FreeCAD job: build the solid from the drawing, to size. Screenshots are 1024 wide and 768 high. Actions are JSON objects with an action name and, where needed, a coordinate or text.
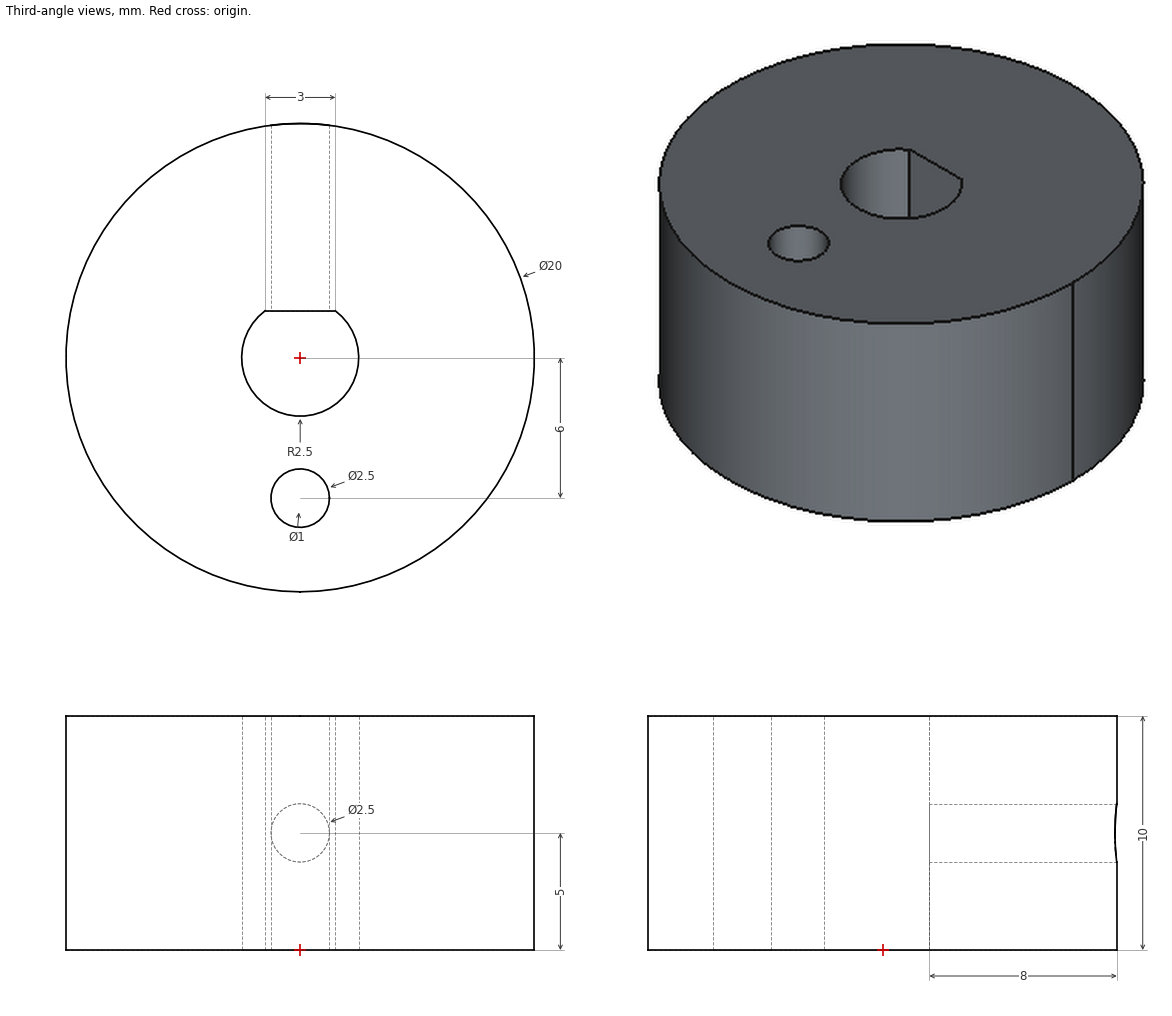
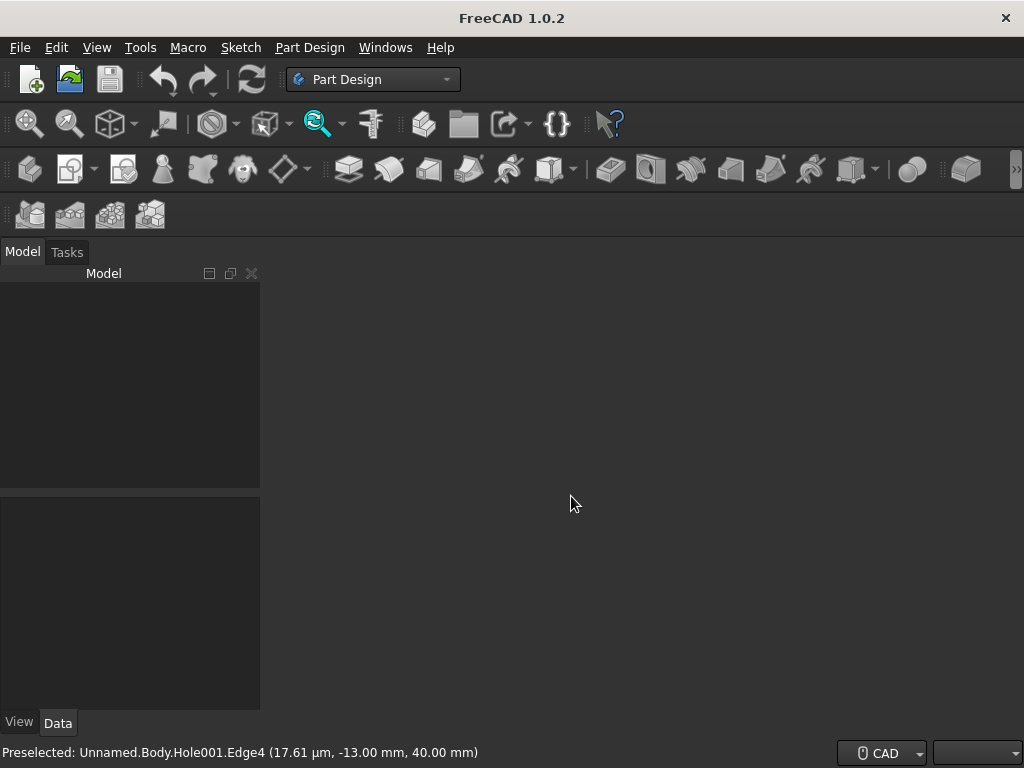
{"action": "left_click", "coordinate": [30, 80]}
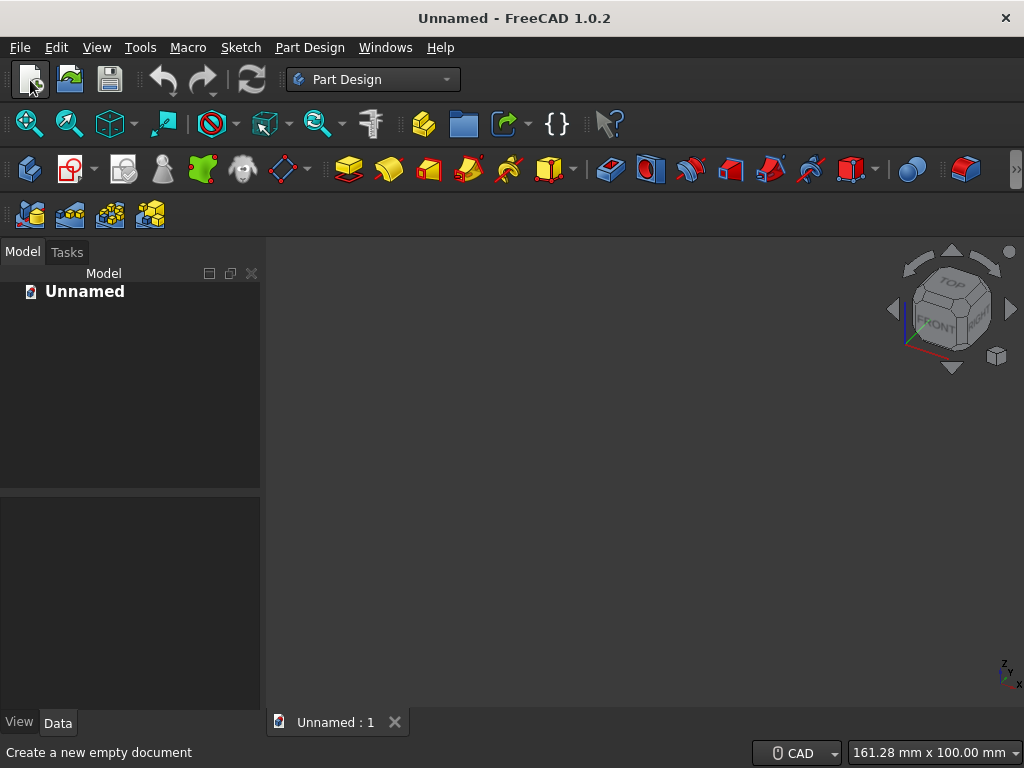
{"action": "left_click", "coordinate": [70, 170]}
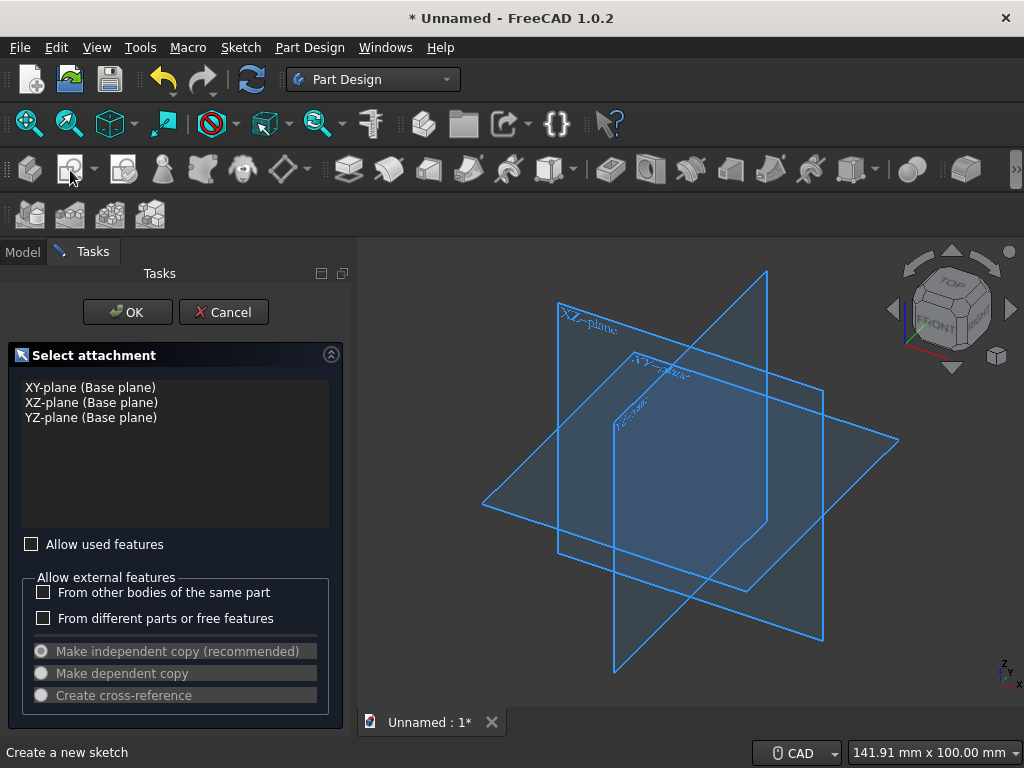
{"action": "left_click", "coordinate": [82, 388]}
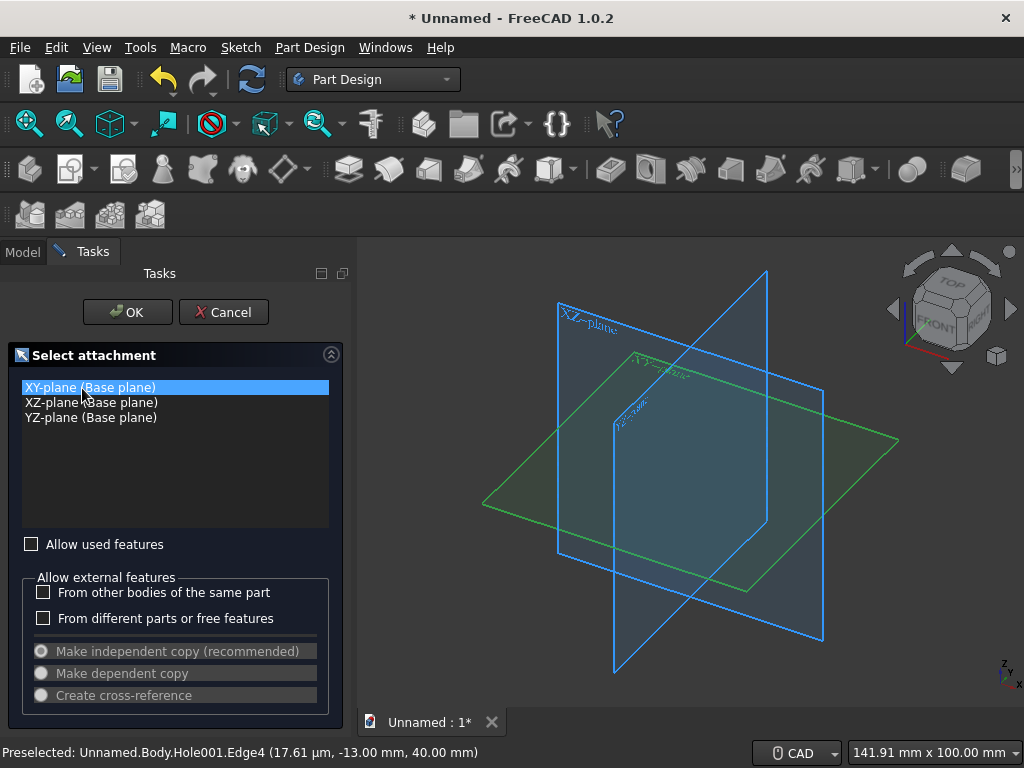
{"action": "left_click", "coordinate": [128, 312]}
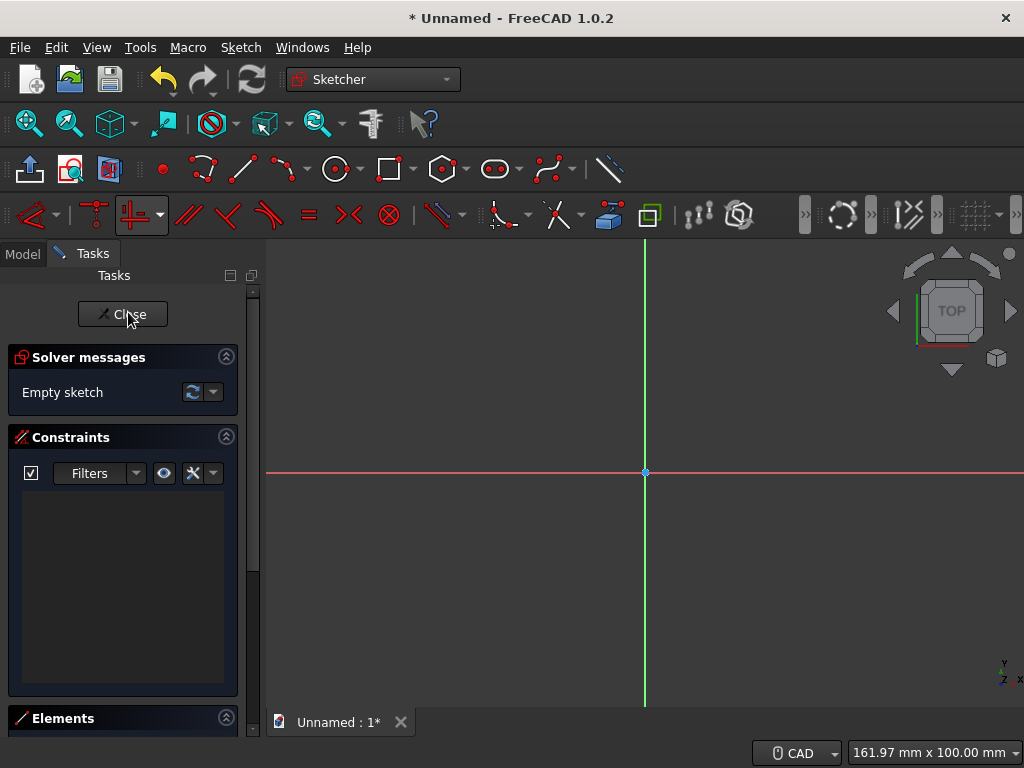
{"action": "scroll", "coordinate": [675, 473], "scroll_direction": "up", "scroll_amount": 6}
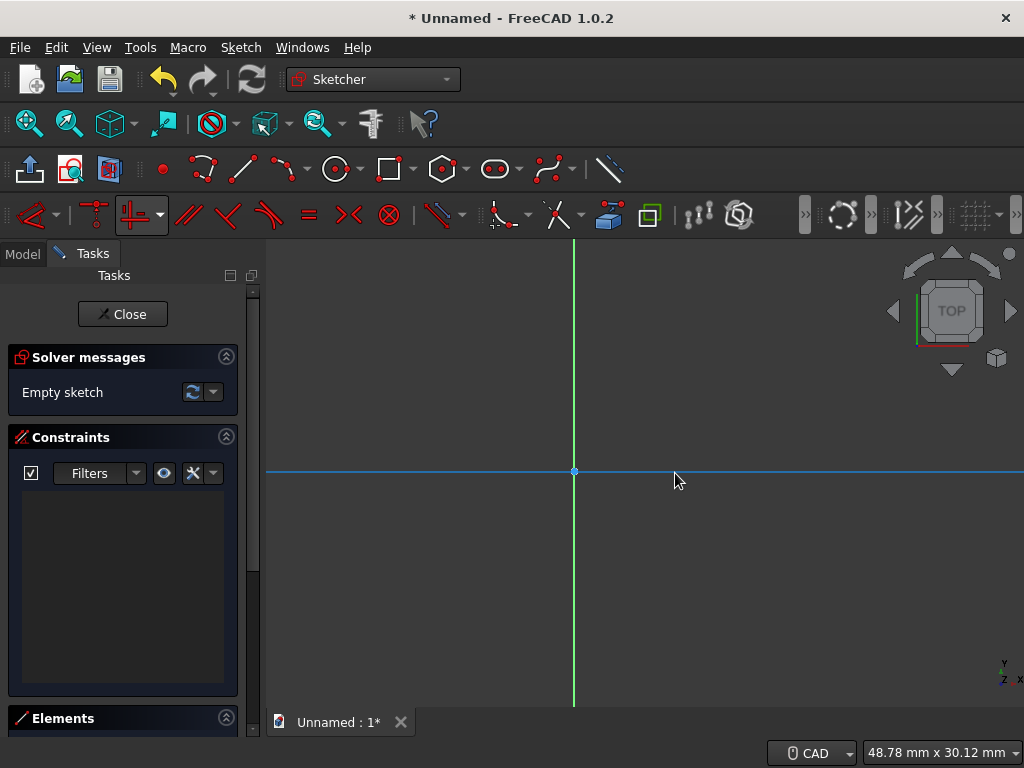
{"action": "left_click", "coordinate": [244, 170]}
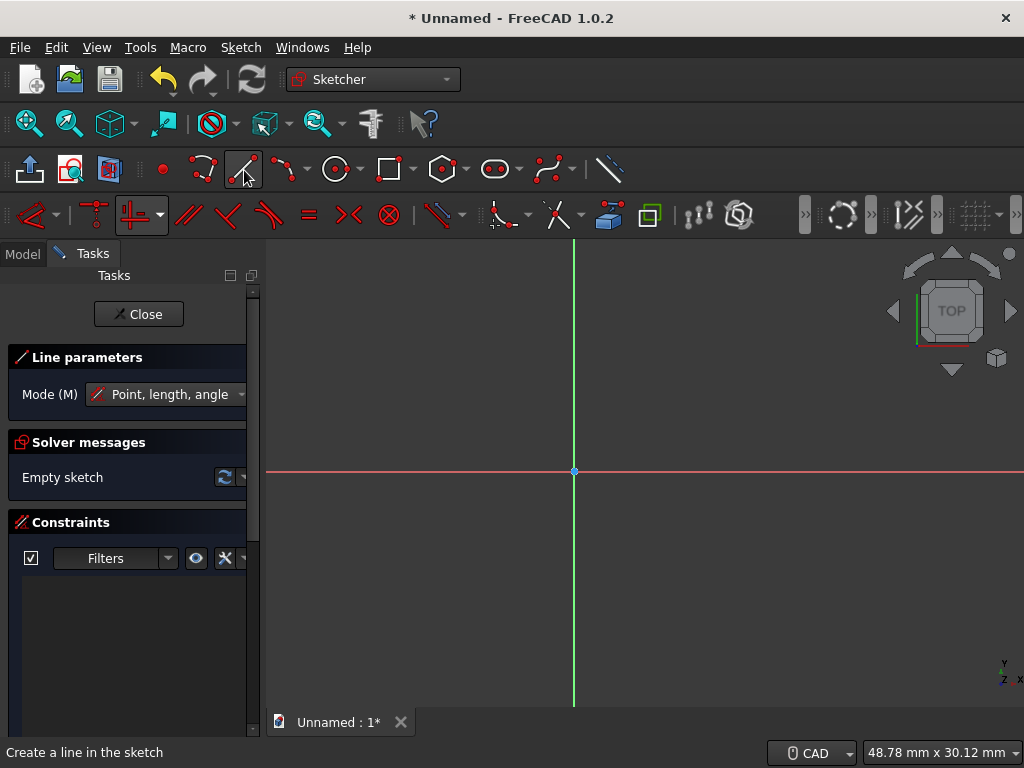
{"action": "left_click", "coordinate": [597, 441]}
{"action": "left_click", "coordinate": [551, 441]}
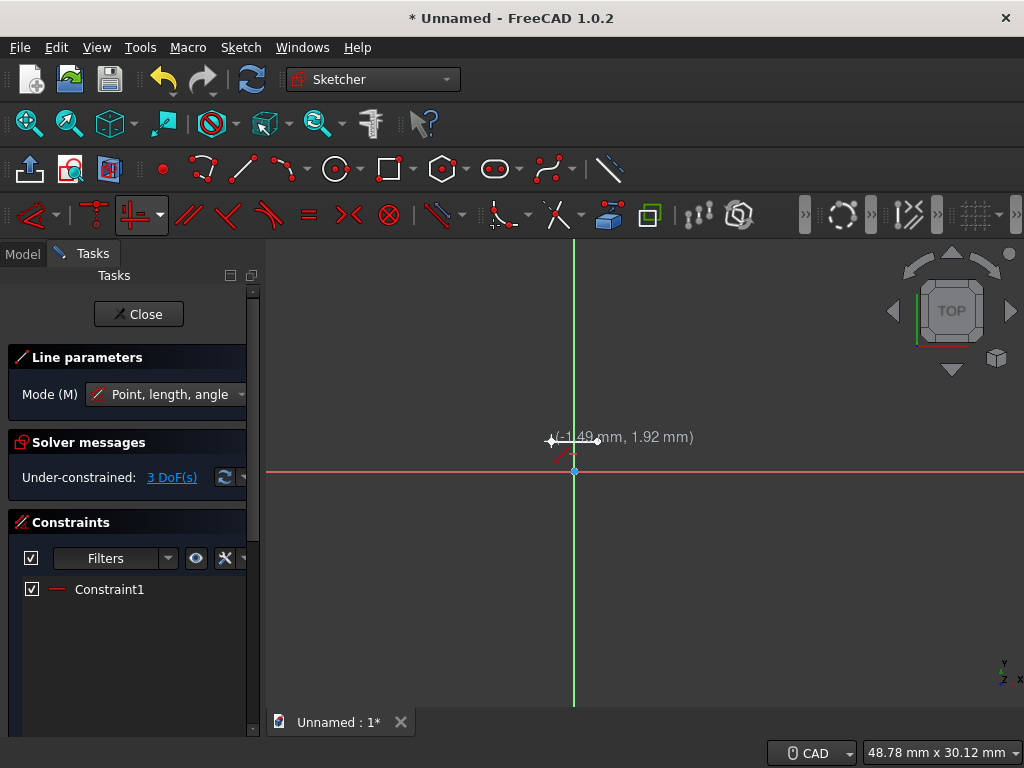
{"action": "left_click", "coordinate": [284, 170]}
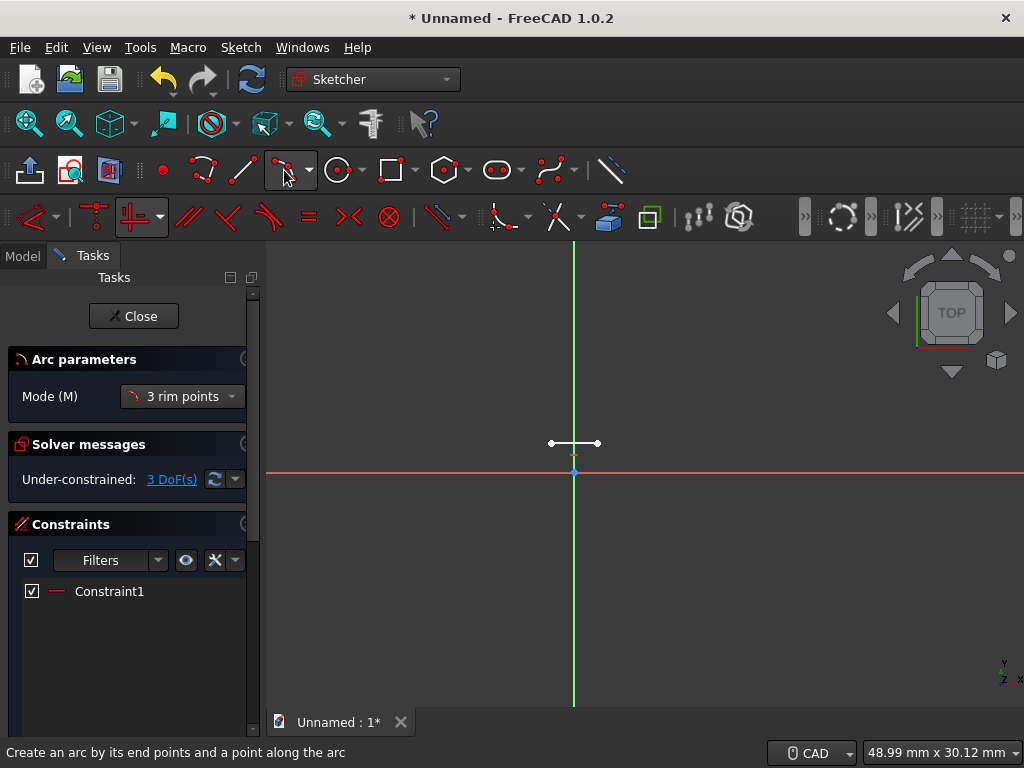
{"action": "left_click", "coordinate": [551, 443]}
{"action": "left_click", "coordinate": [597, 443]}
{"action": "left_click", "coordinate": [556, 507]}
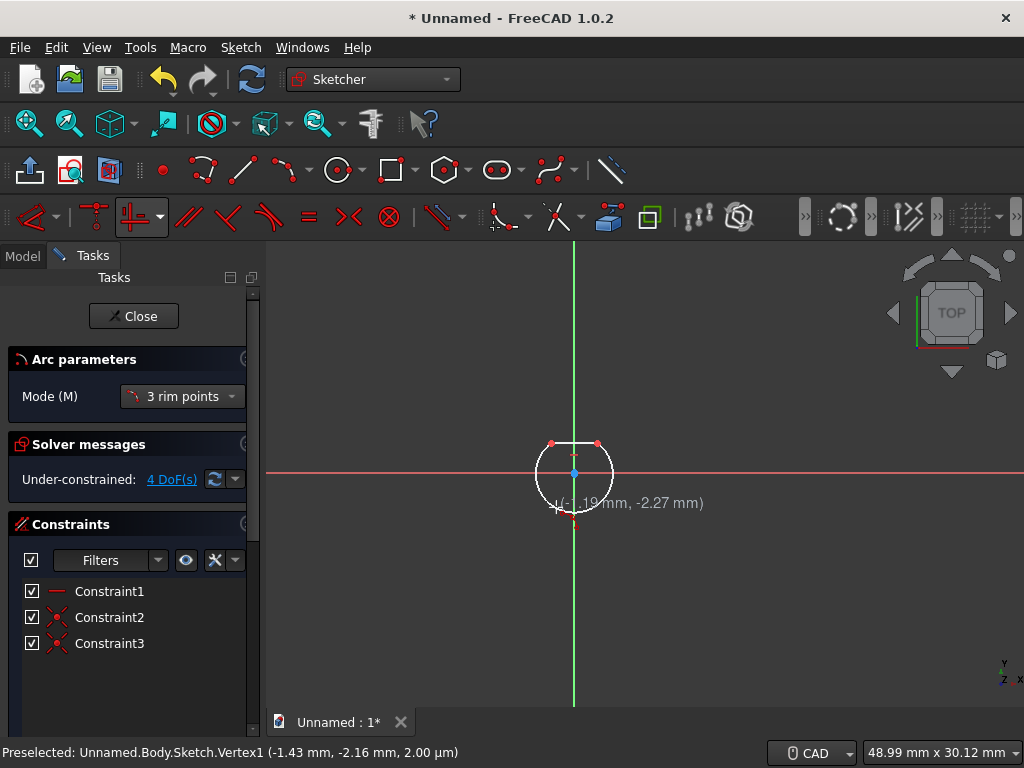
{"action": "left_click", "coordinate": [338, 170]}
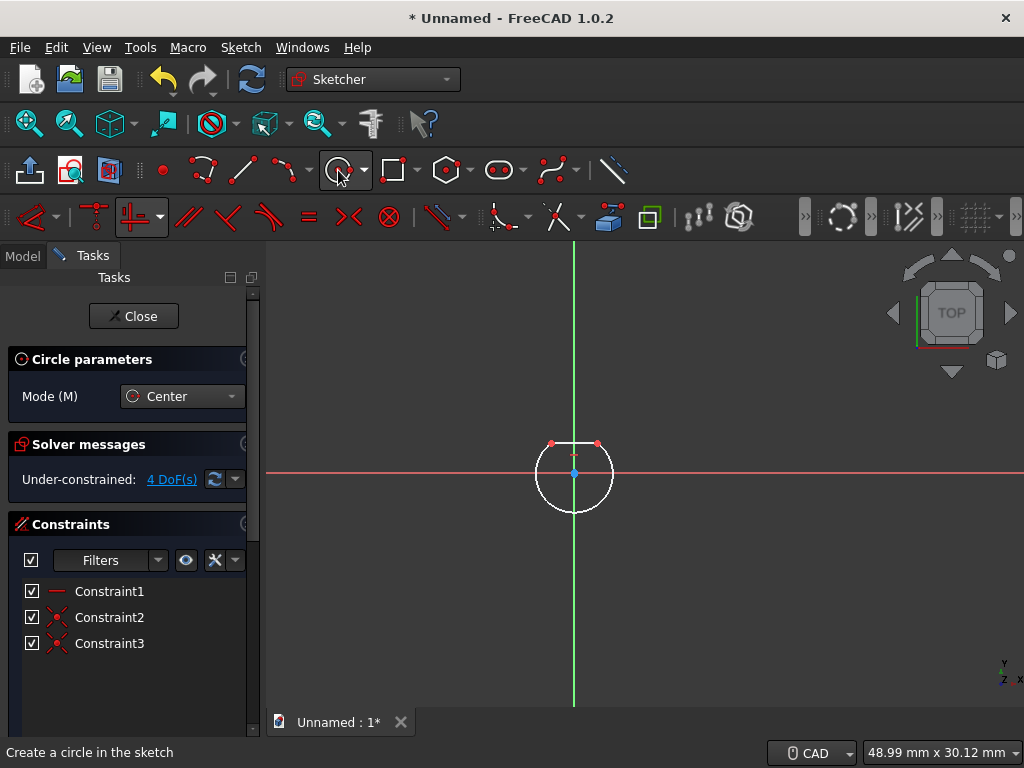
{"action": "left_click", "coordinate": [574, 473]}
{"action": "mouse_move", "coordinate": [684, 363]}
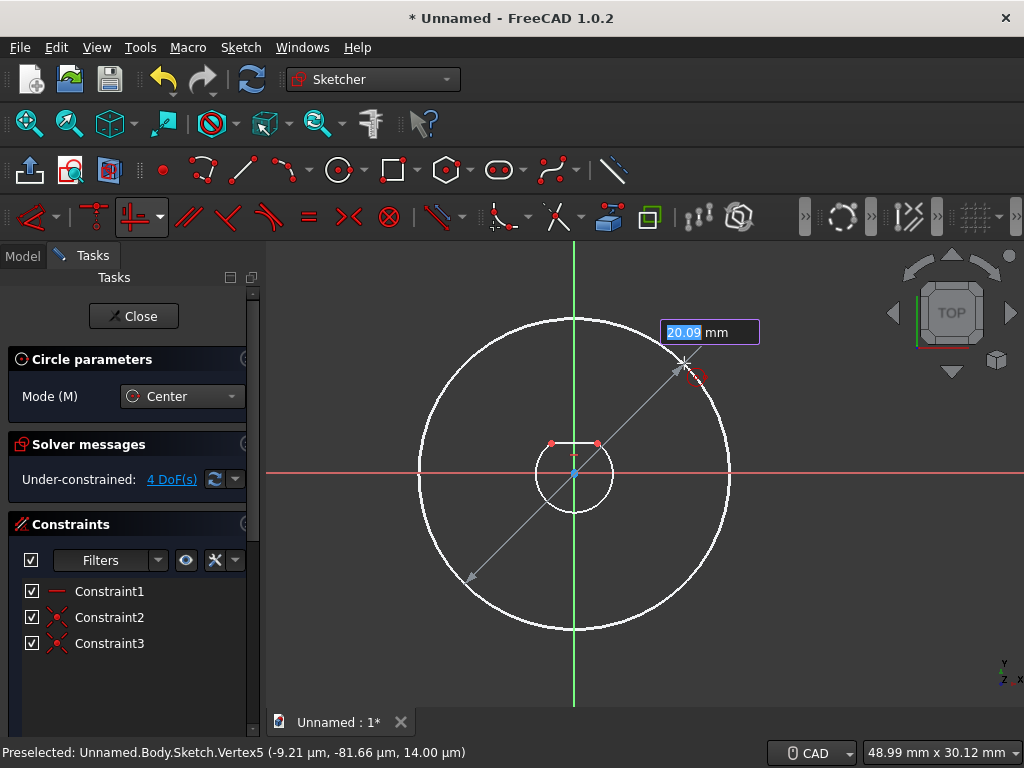
{"action": "type", "text": "20"}
{"action": "key", "text": "Return"}
{"action": "key", "text": "Escape"}